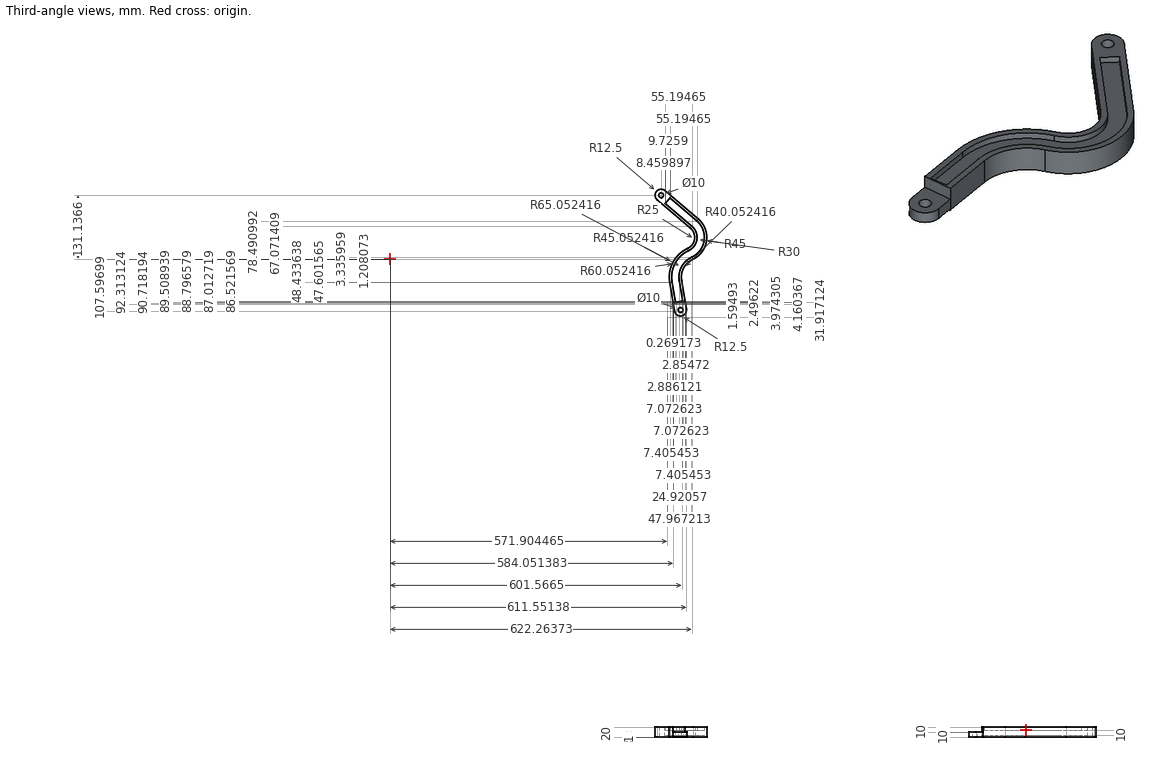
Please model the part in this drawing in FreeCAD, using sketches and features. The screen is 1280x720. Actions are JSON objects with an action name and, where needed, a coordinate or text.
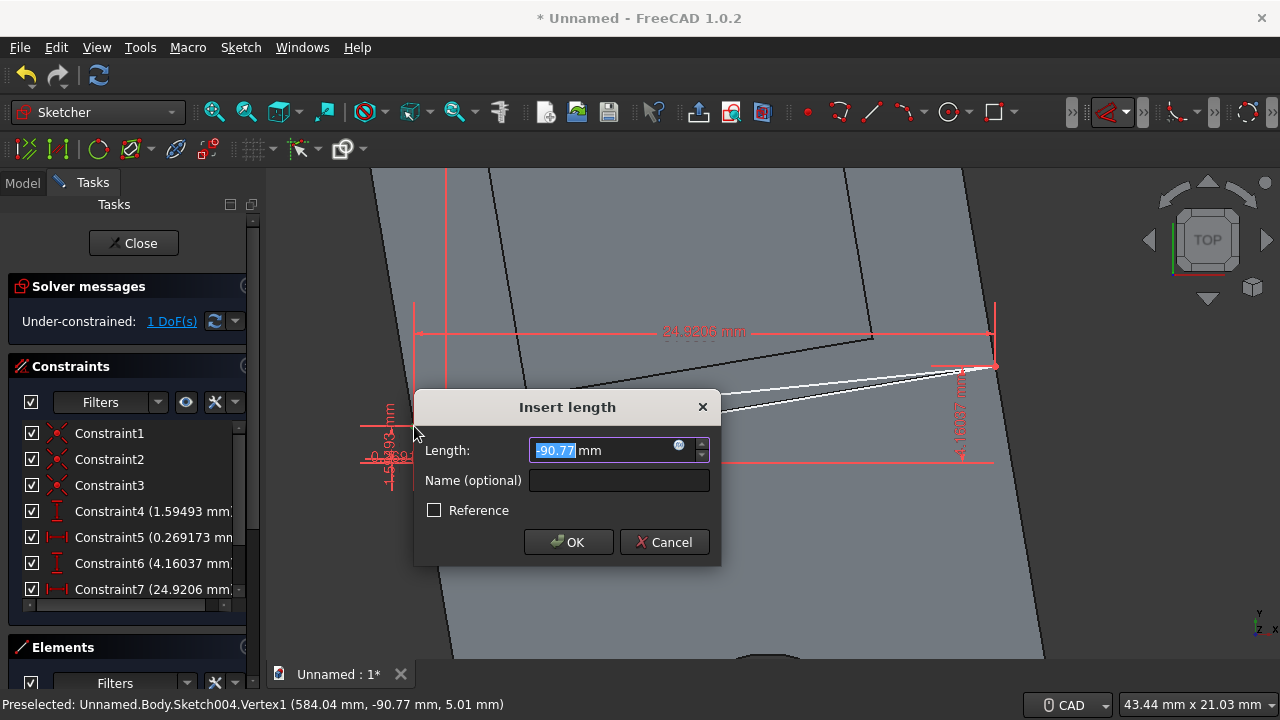
{"action": "type", "text": "-90.718194"}
{"action": "key", "text": "Return"}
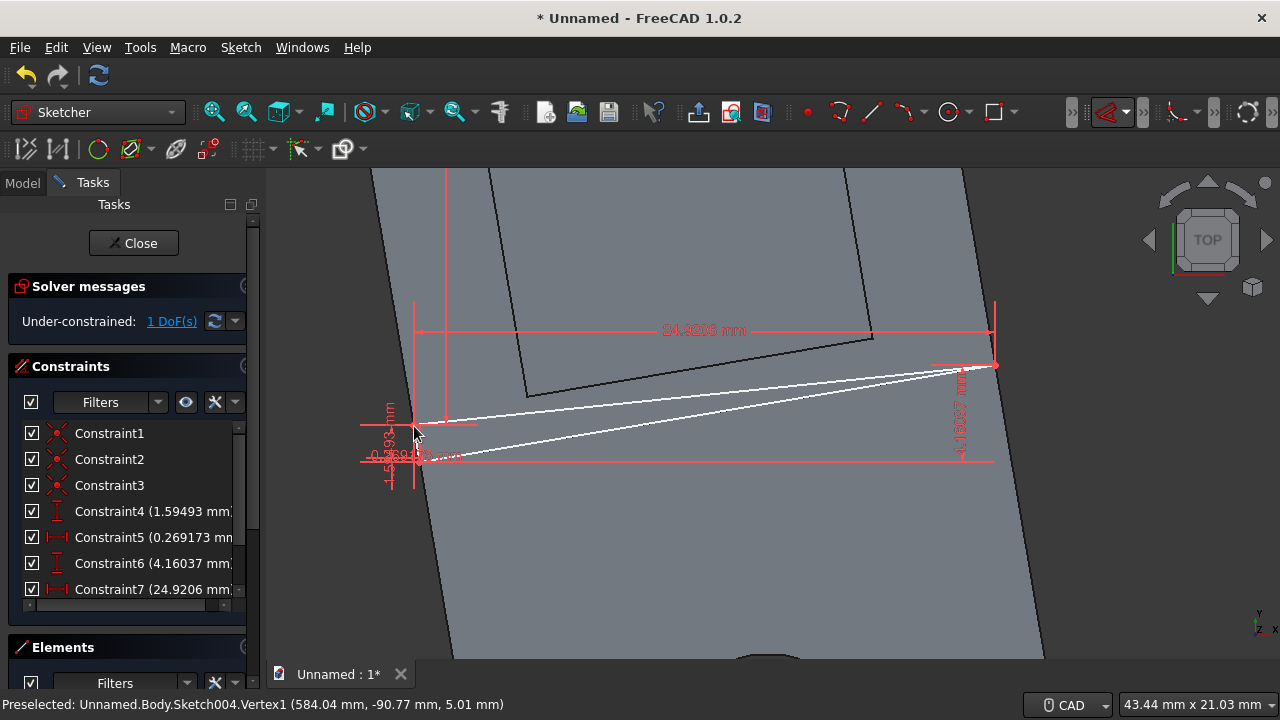
{"action": "left_click", "coordinate": [414, 425]}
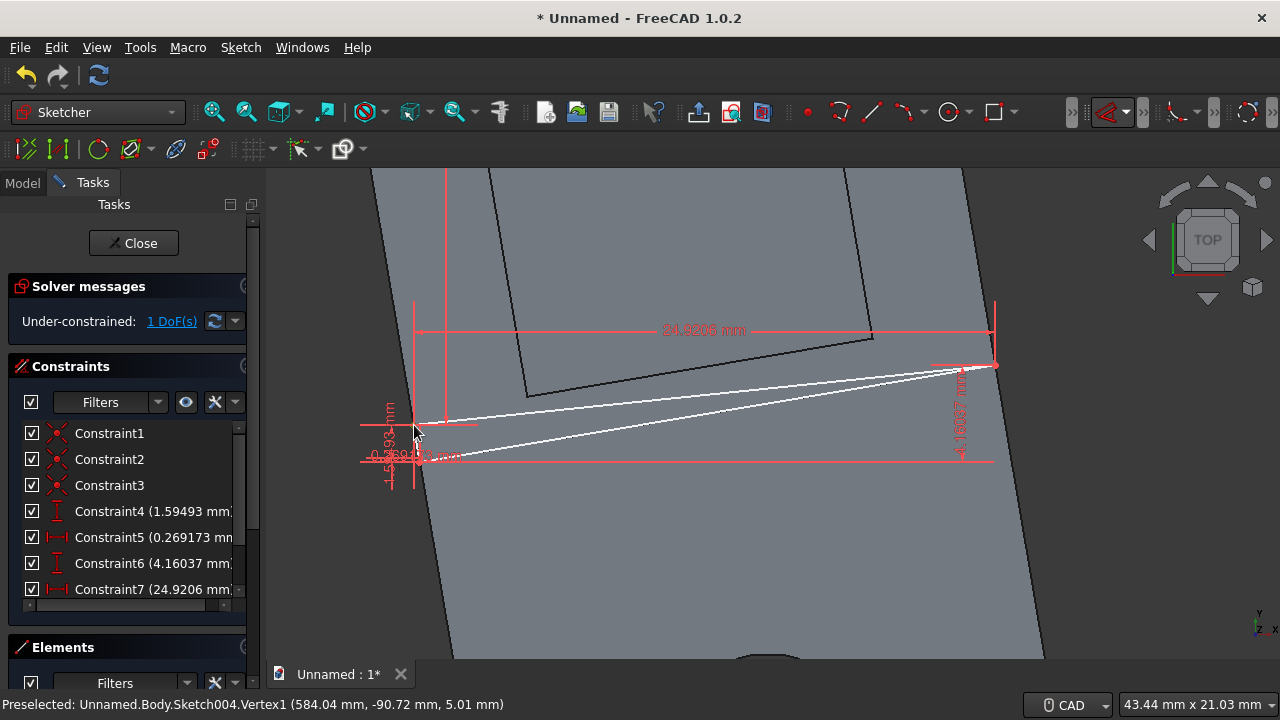
{"action": "key", "text": "l"}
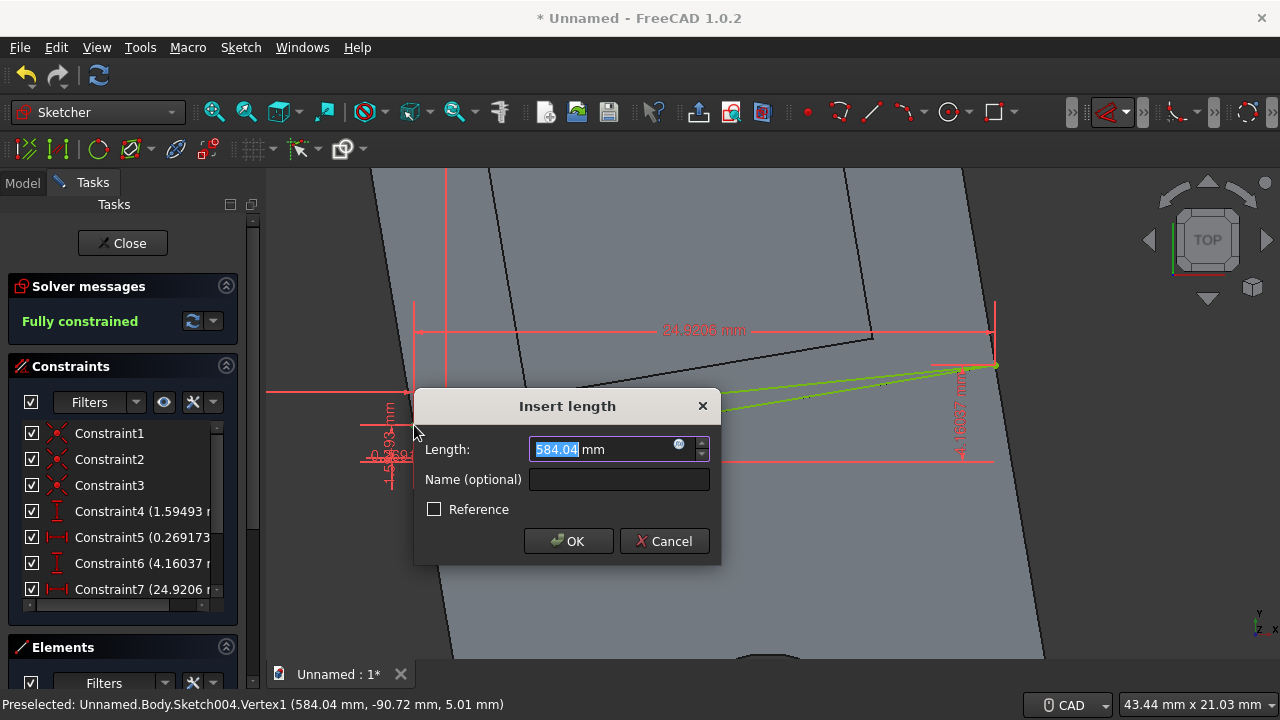
{"action": "type", "text": "584.051383"}
{"action": "key", "text": "Return"}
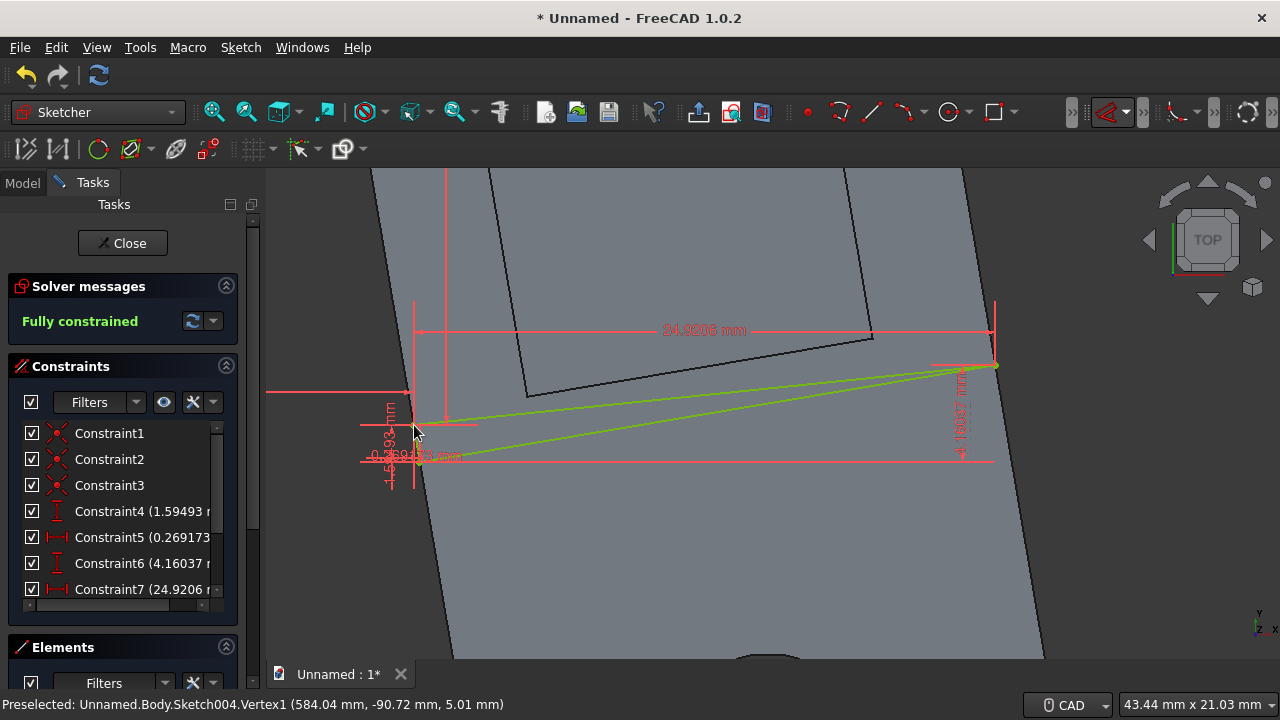
{"action": "left_click", "coordinate": [123, 243]}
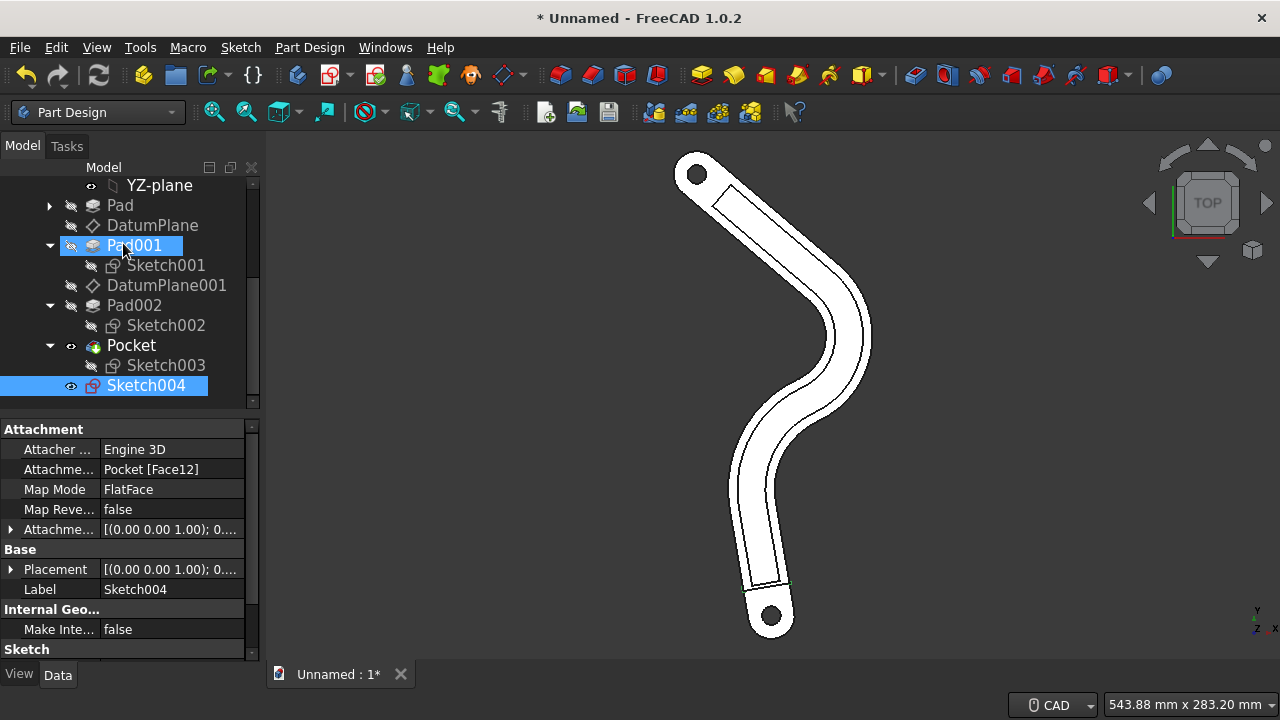
{"action": "left_click", "coordinate": [916, 76]}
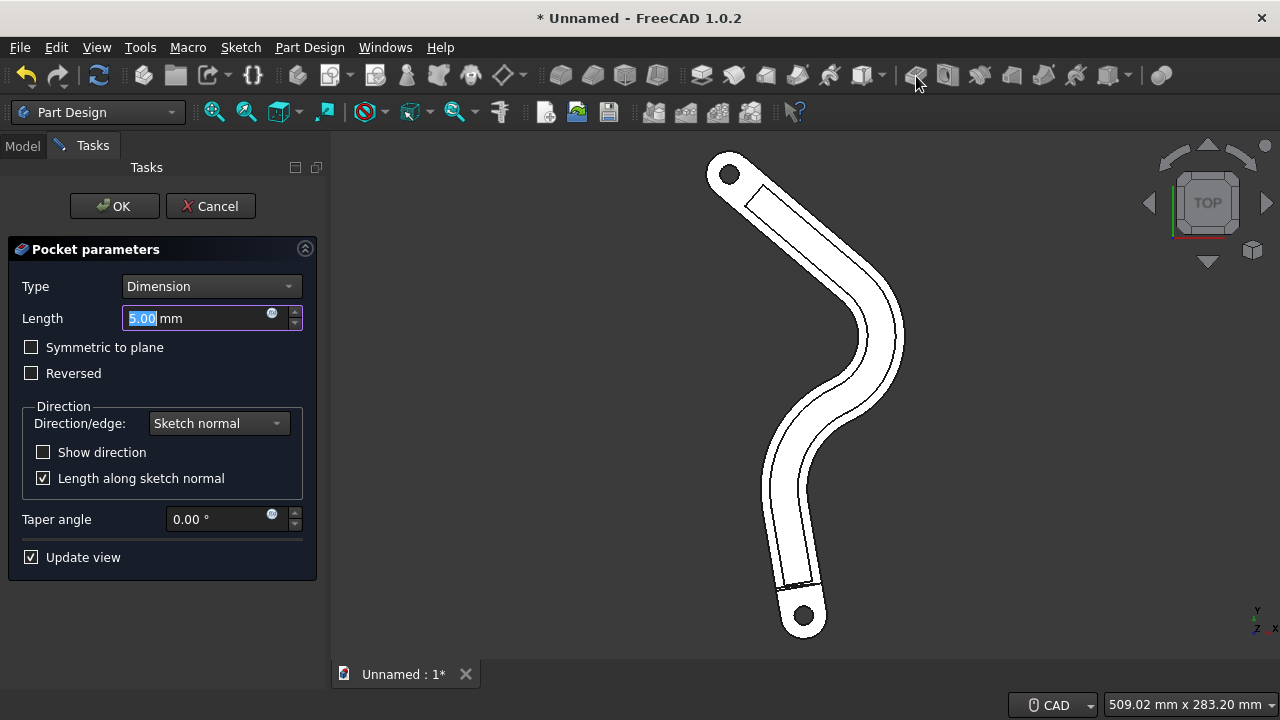
{"action": "type", "text": "10"}
{"action": "key", "text": "Tab"}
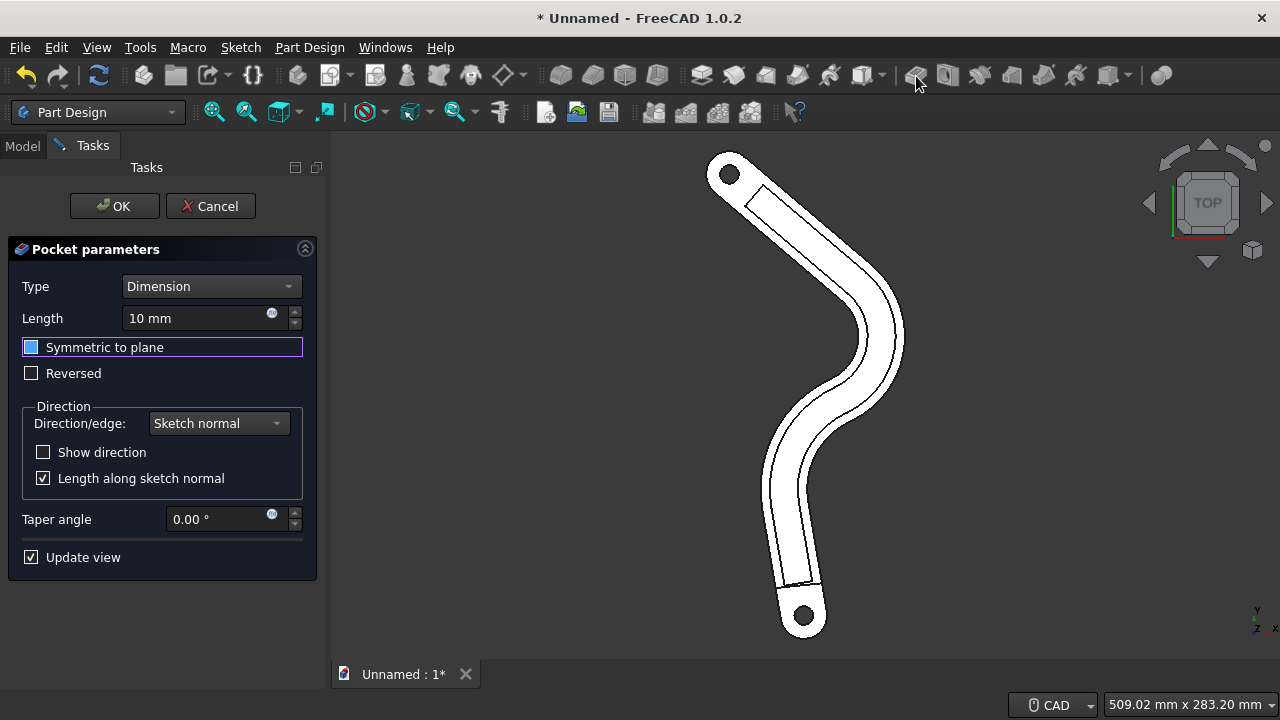
{"action": "left_click", "coordinate": [115, 206]}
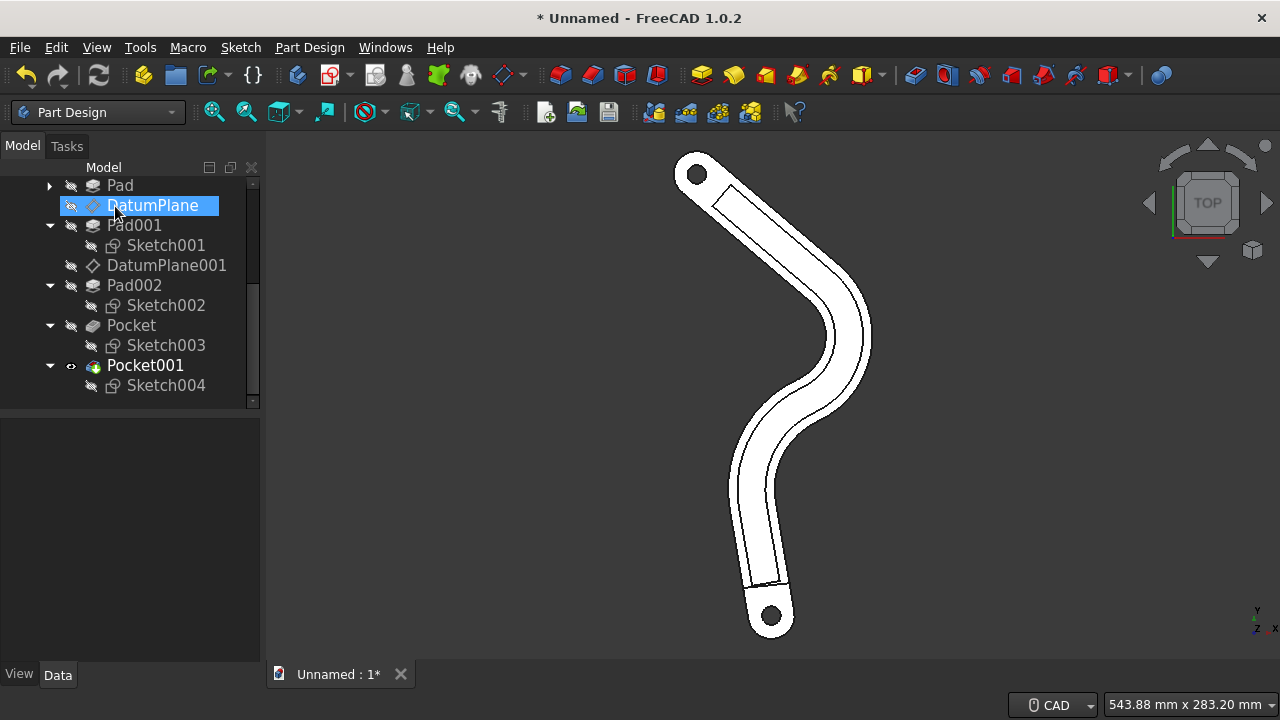
{"action": "key", "text": "0"}